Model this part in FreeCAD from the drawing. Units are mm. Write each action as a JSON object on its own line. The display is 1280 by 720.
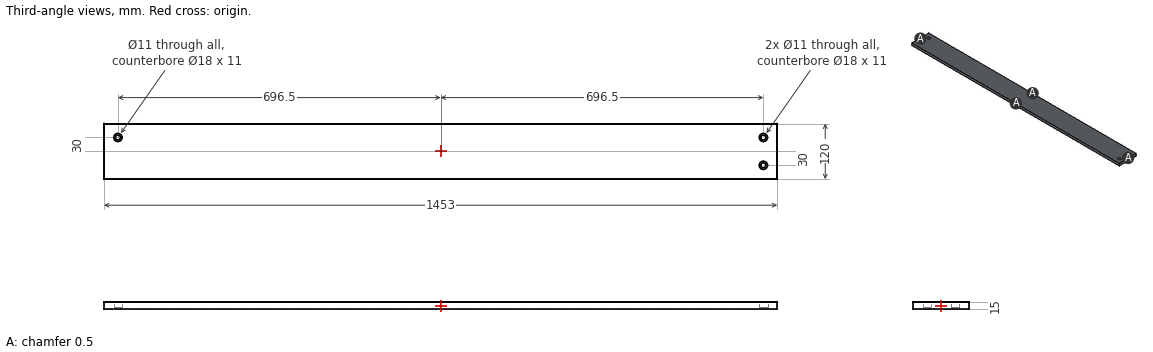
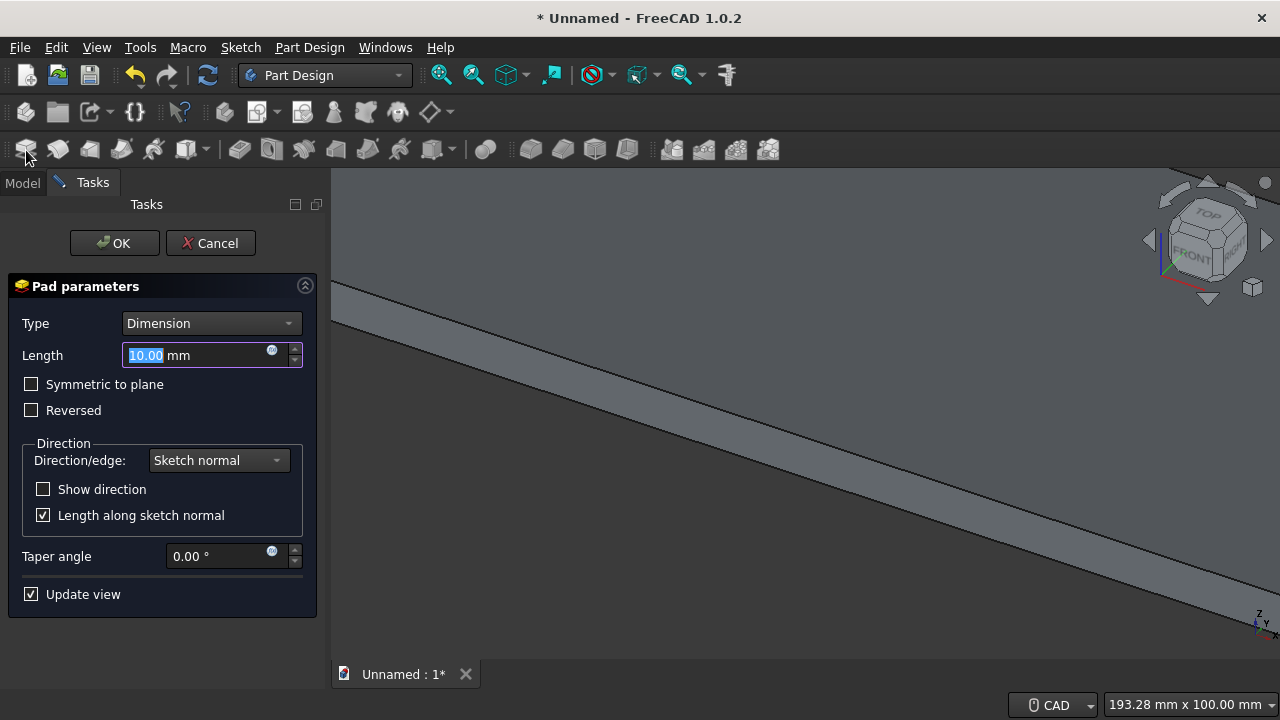
{"action": "type", "text": "15"}
{"action": "key", "text": "Tab"}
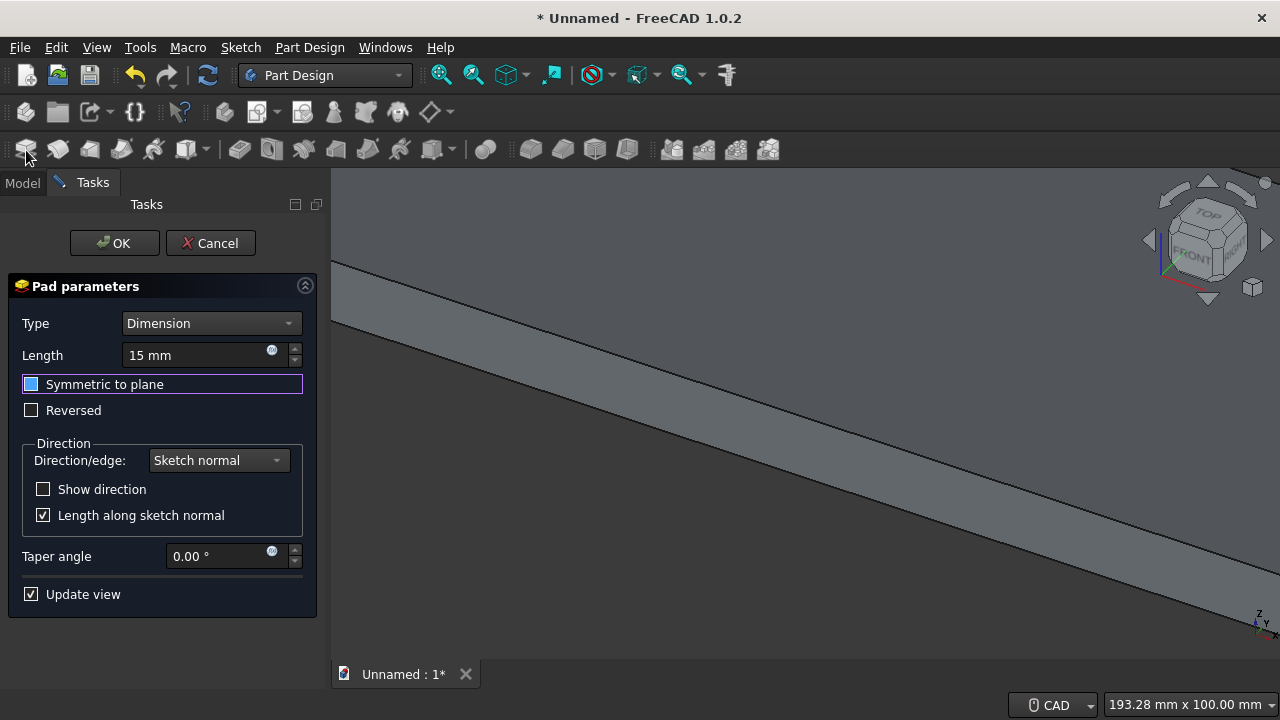
{"action": "left_click", "coordinate": [30, 384]}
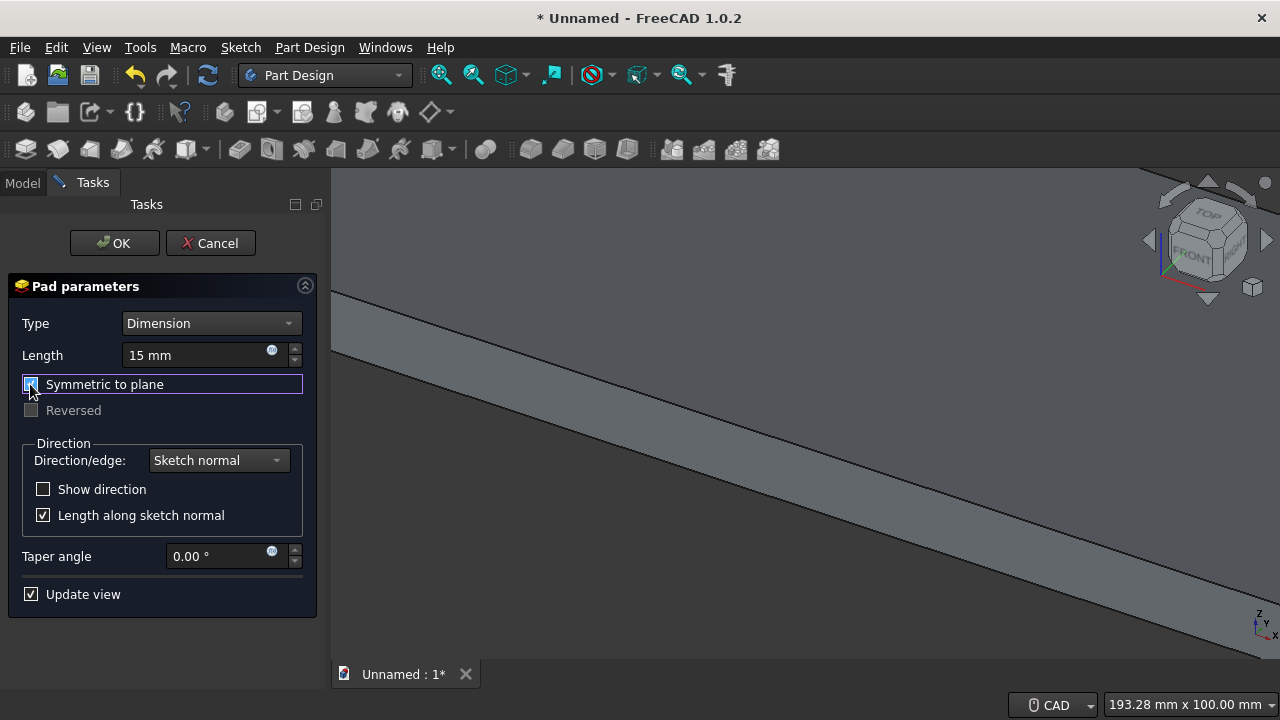
{"action": "left_click", "coordinate": [115, 243]}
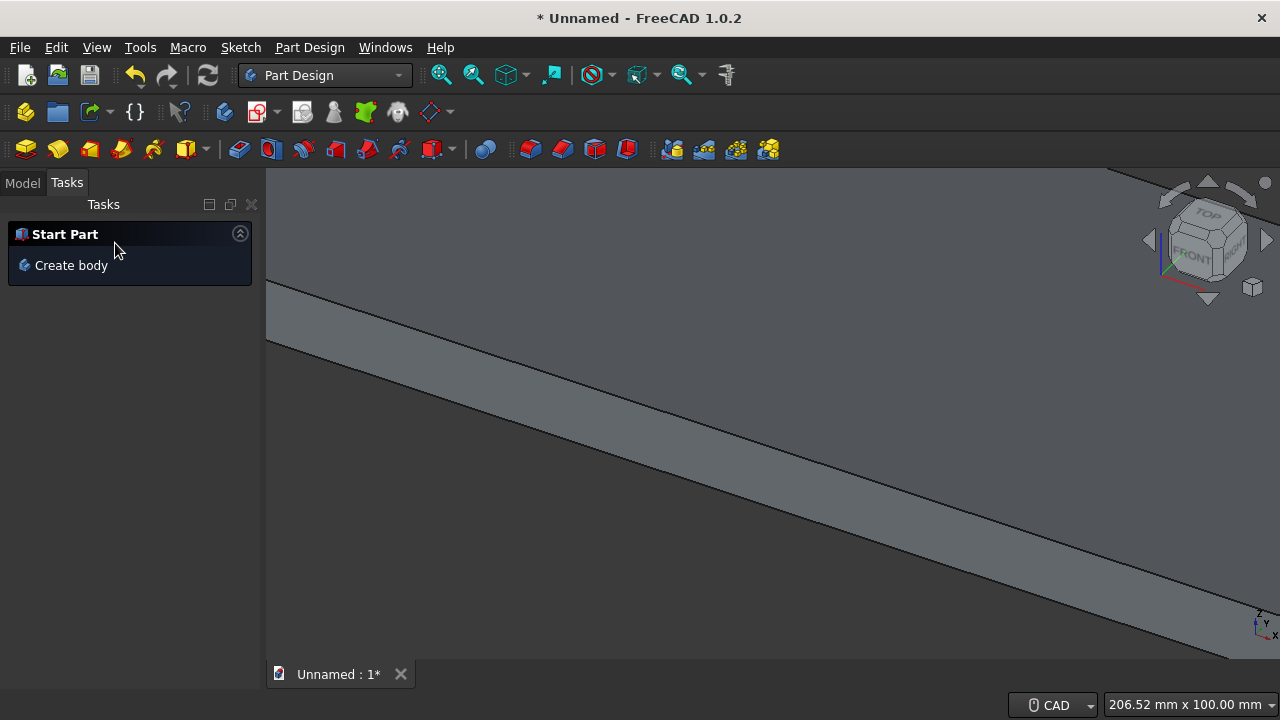
{"action": "key", "text": "v f"}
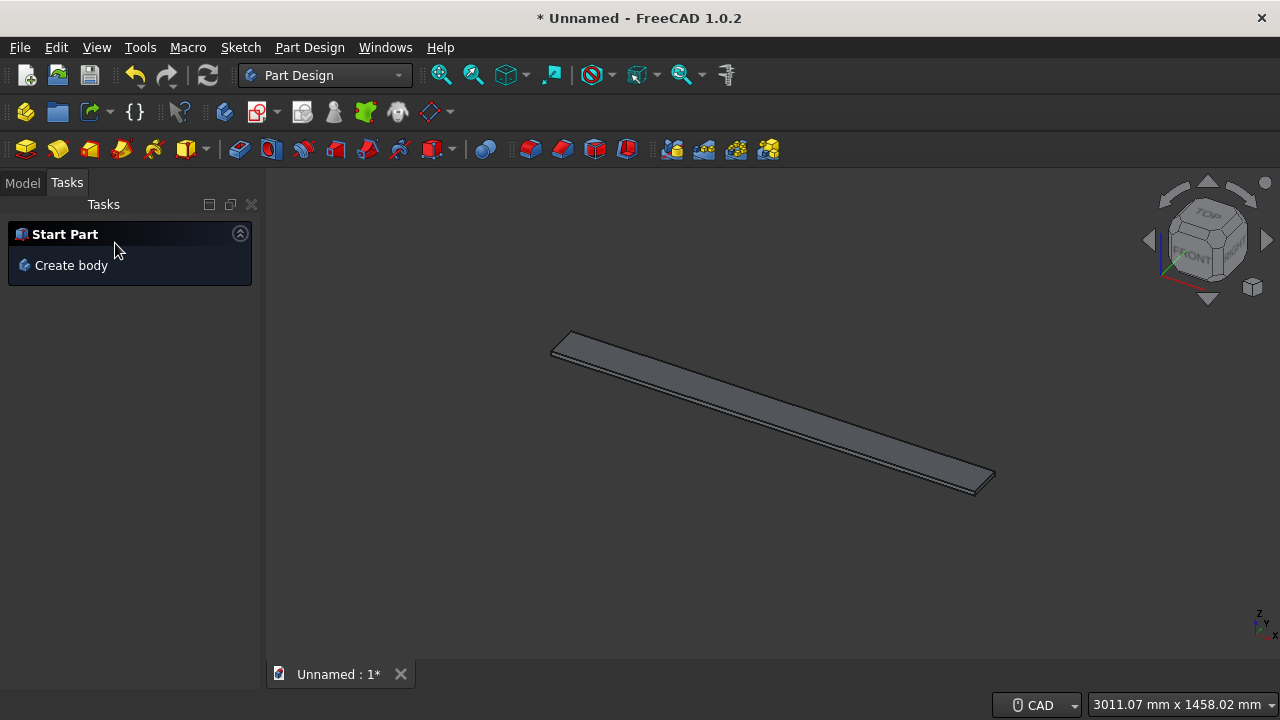
{"action": "left_click", "coordinate": [955, 471]}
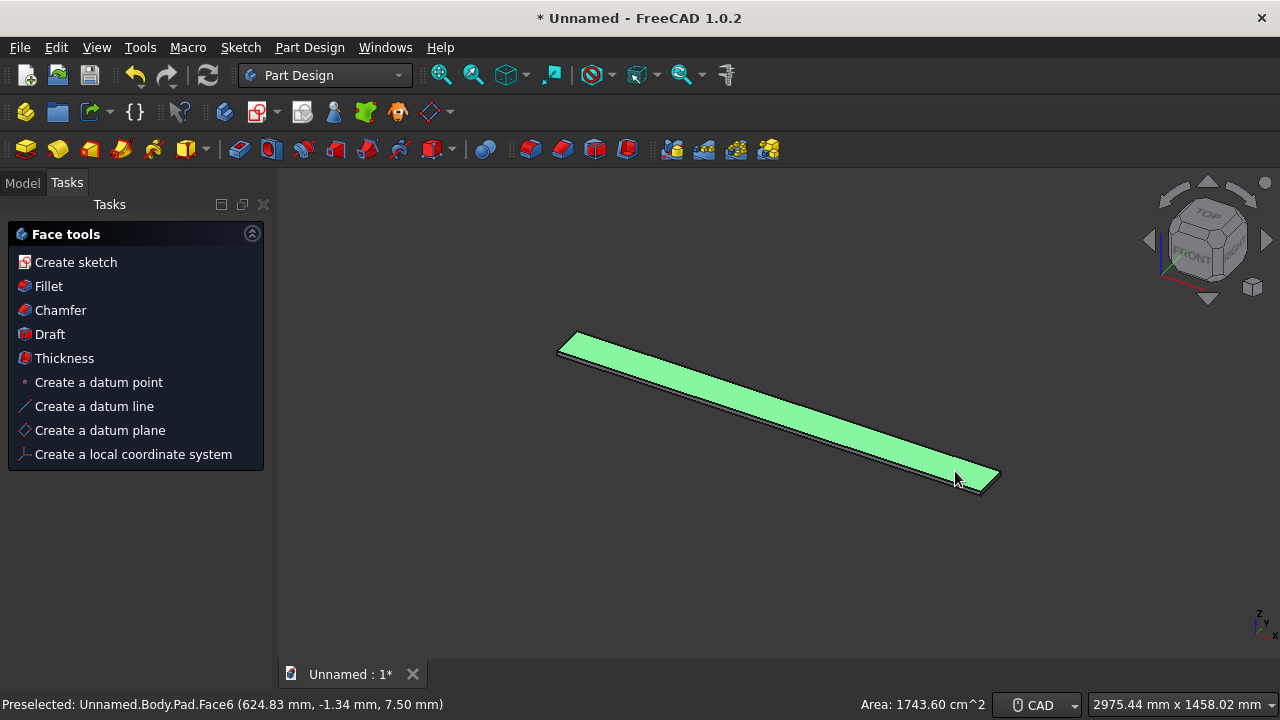
{"action": "left_click", "coordinate": [258, 112]}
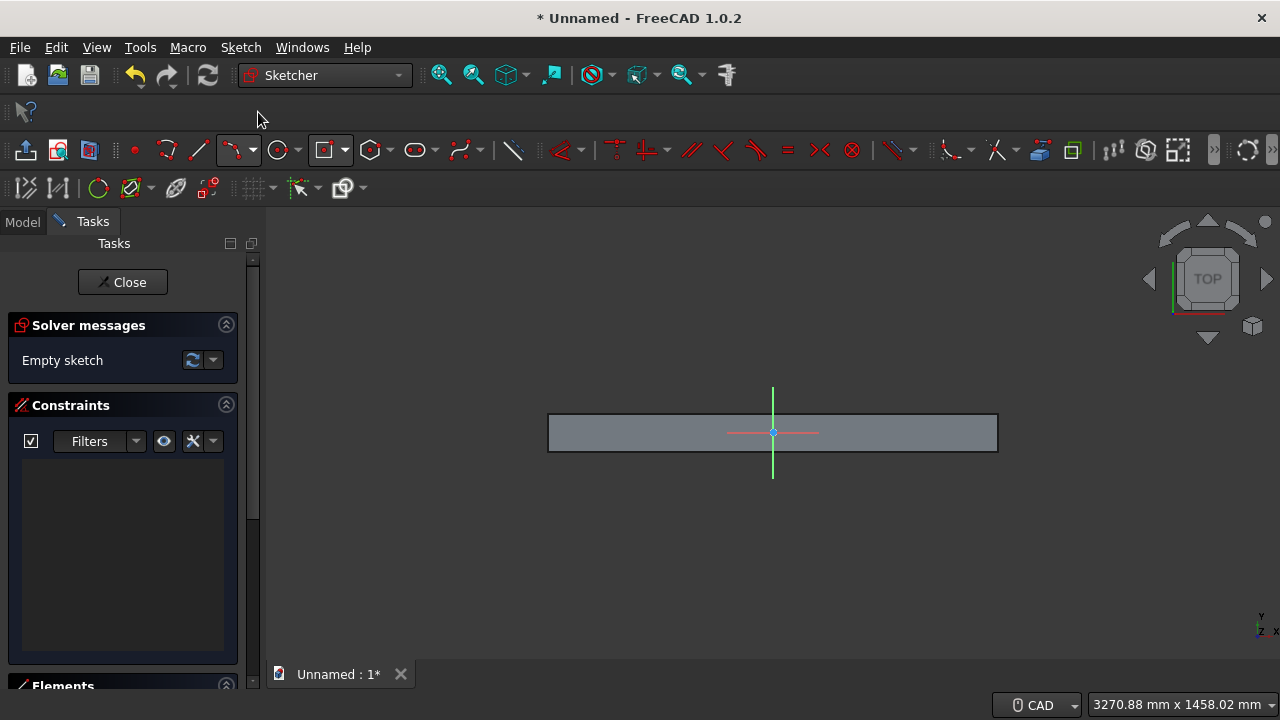
{"action": "scroll", "coordinate": [549, 423], "scroll_direction": "up", "scroll_amount": 15}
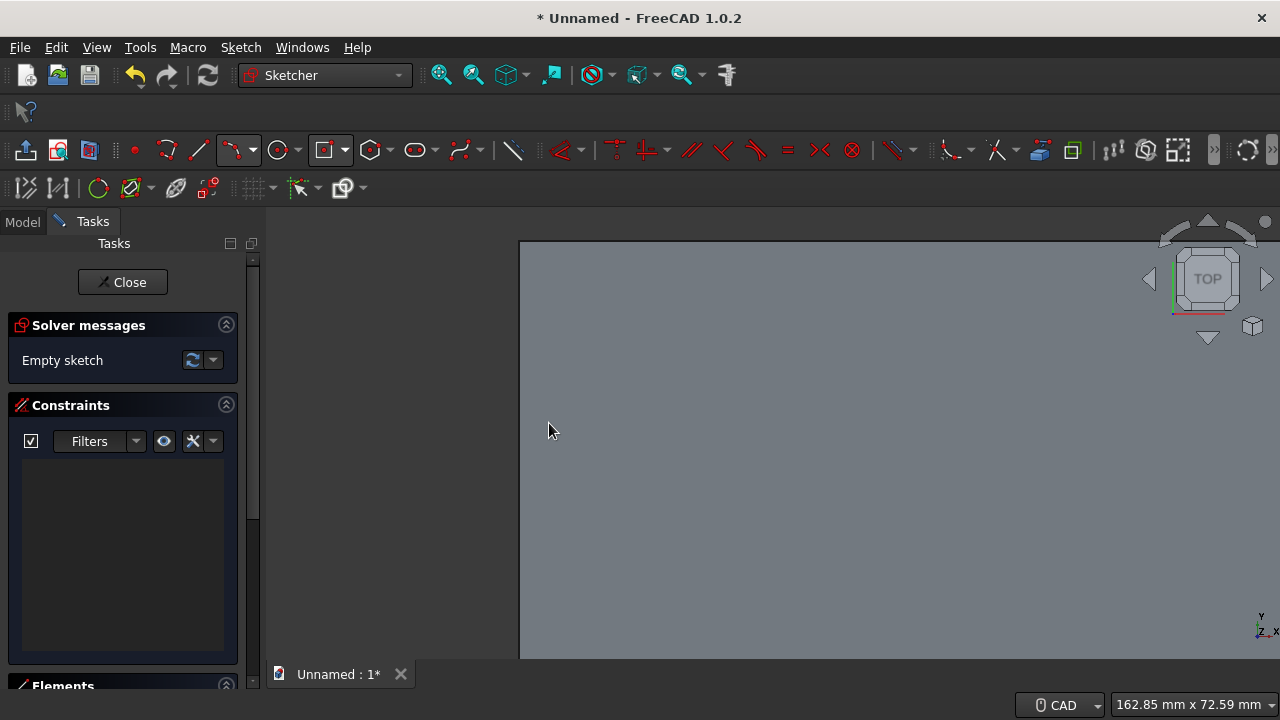
{"action": "scroll", "coordinate": [706, 426], "scroll_direction": "up", "scroll_amount": 7}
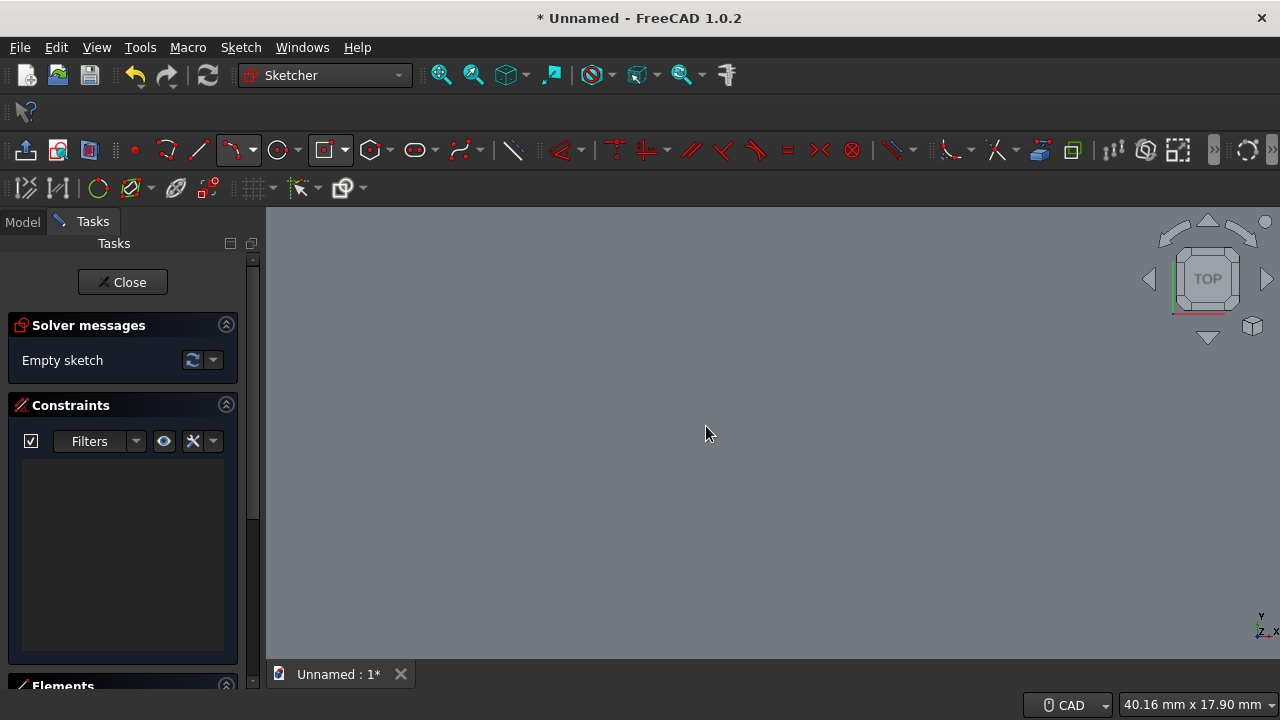
{"action": "left_click", "coordinate": [278, 150]}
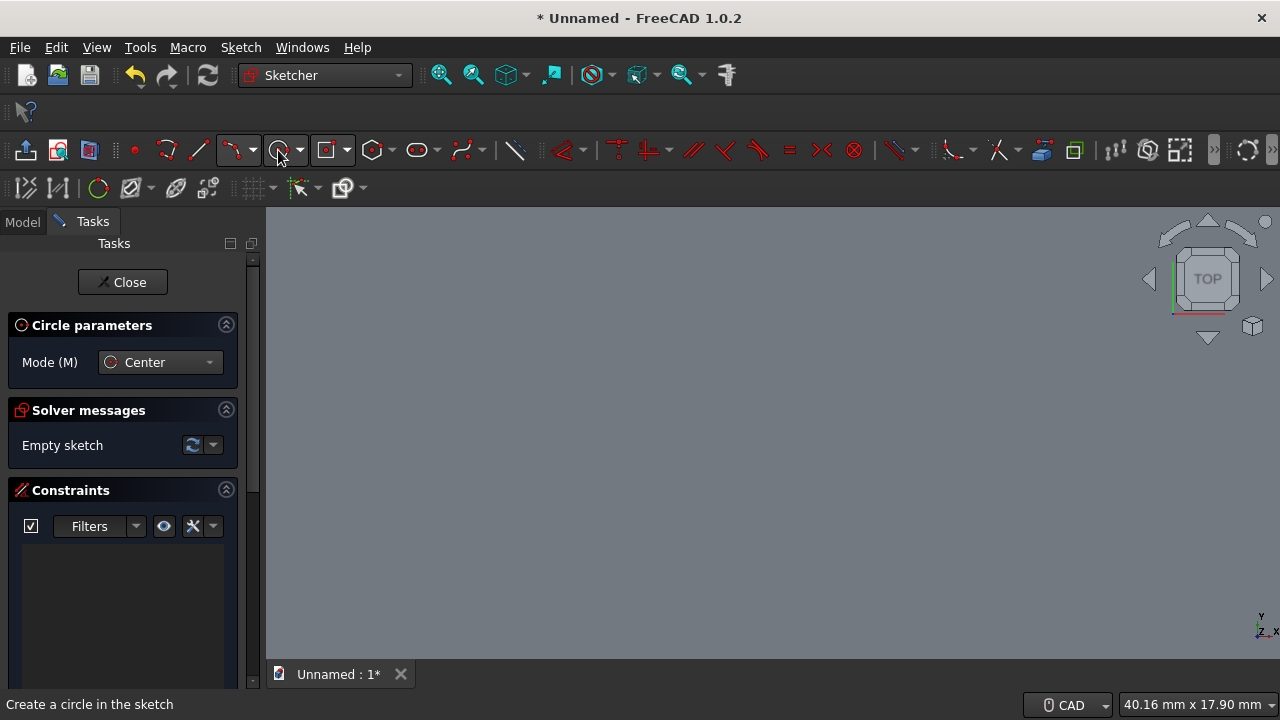
{"action": "left_click", "coordinate": [704, 432]}
{"action": "mouse_move", "coordinate": [803, 334]}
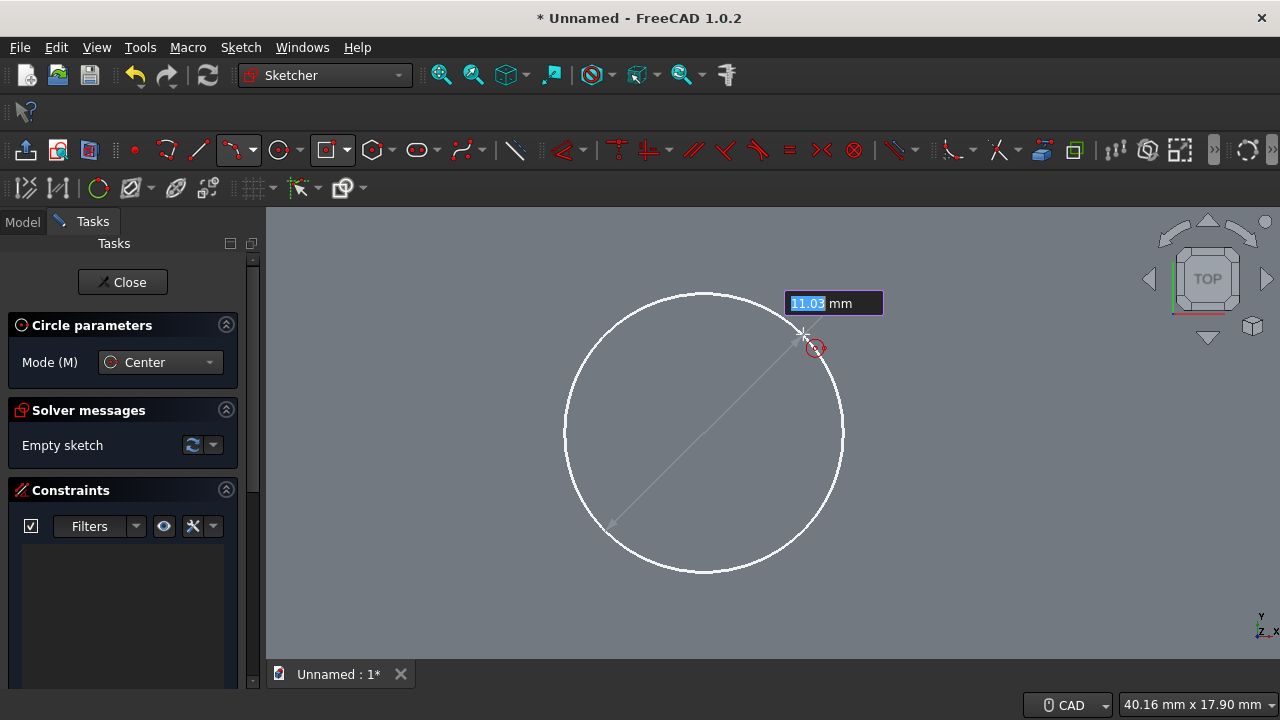
{"action": "type", "text": "11"}
{"action": "key", "text": "Return"}
{"action": "key", "text": "Escape"}